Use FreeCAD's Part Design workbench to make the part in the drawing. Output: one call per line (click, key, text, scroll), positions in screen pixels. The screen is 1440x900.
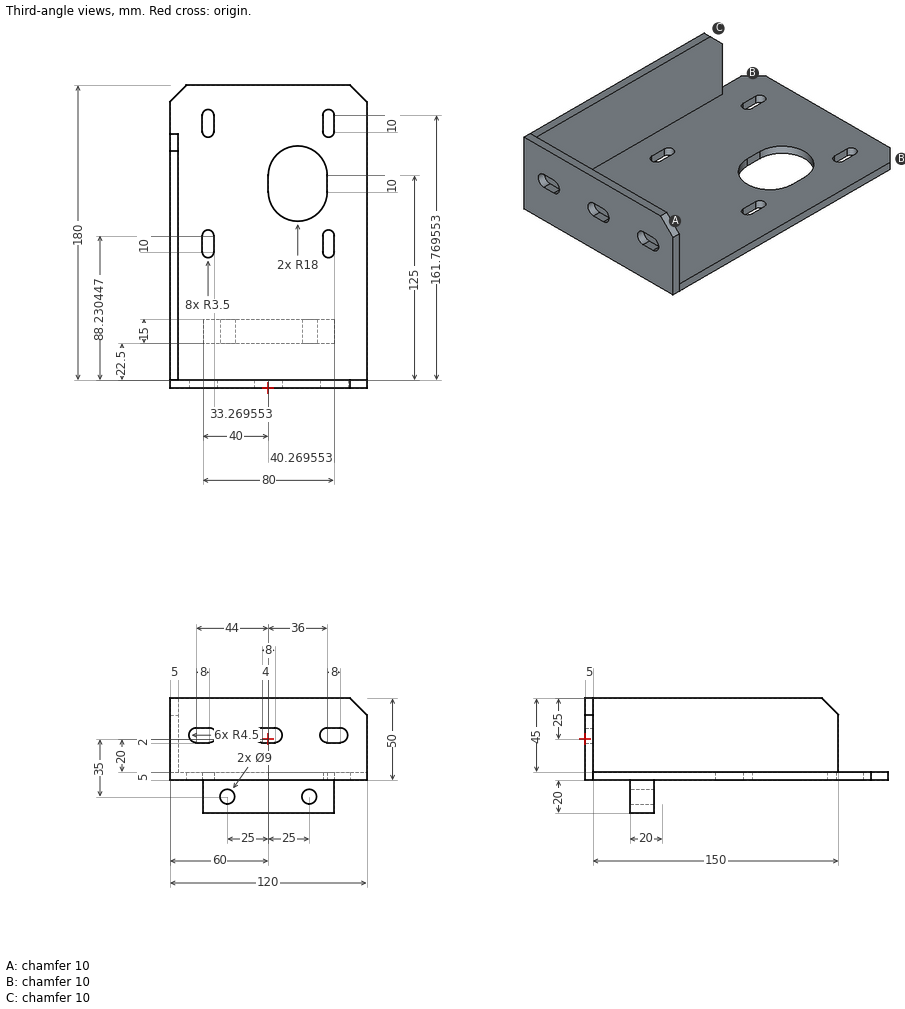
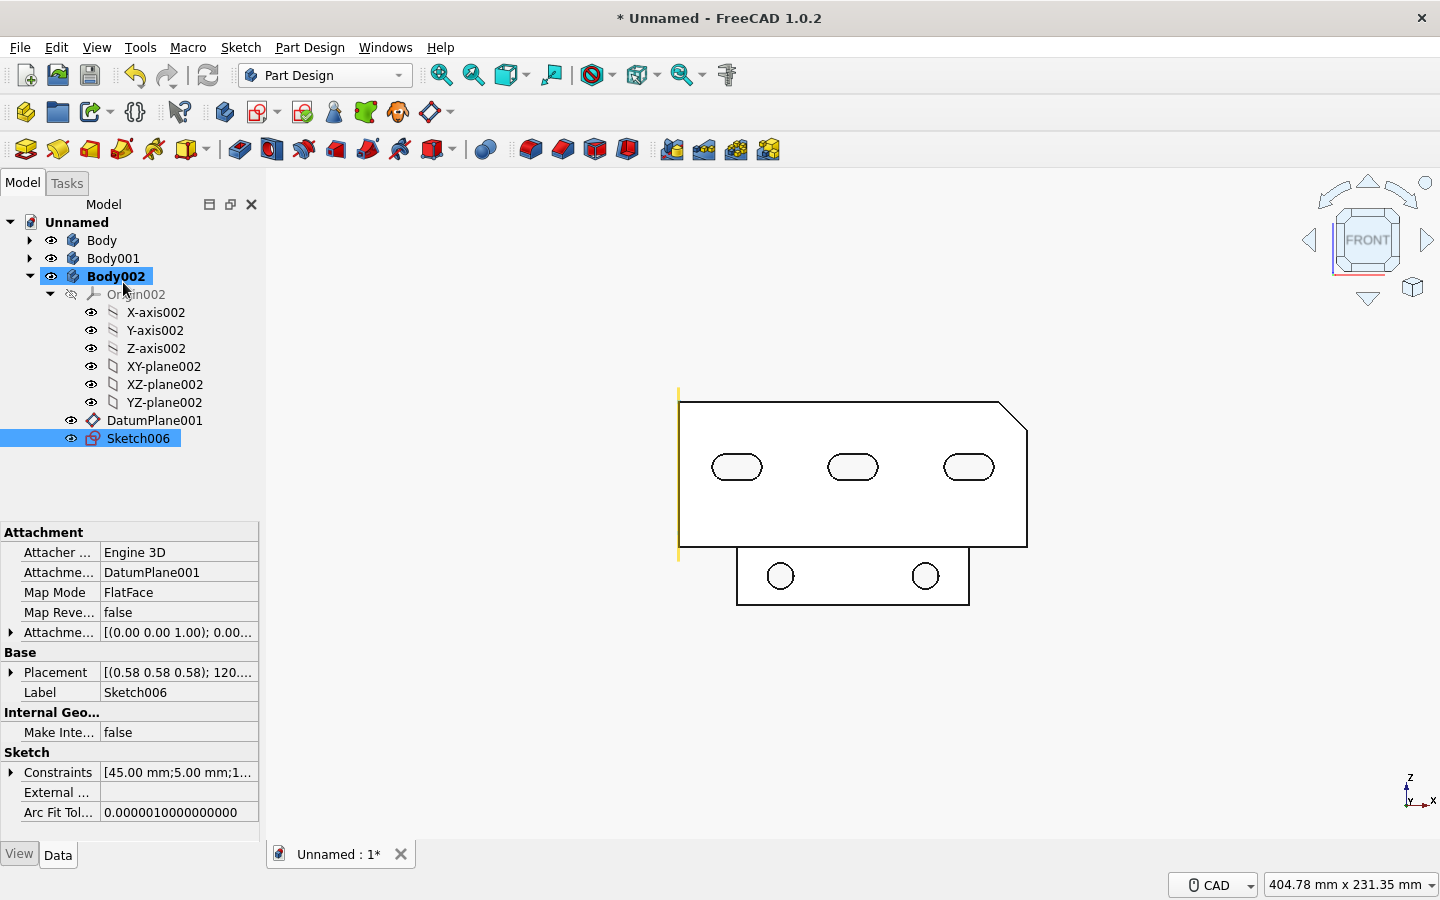
click(26, 150)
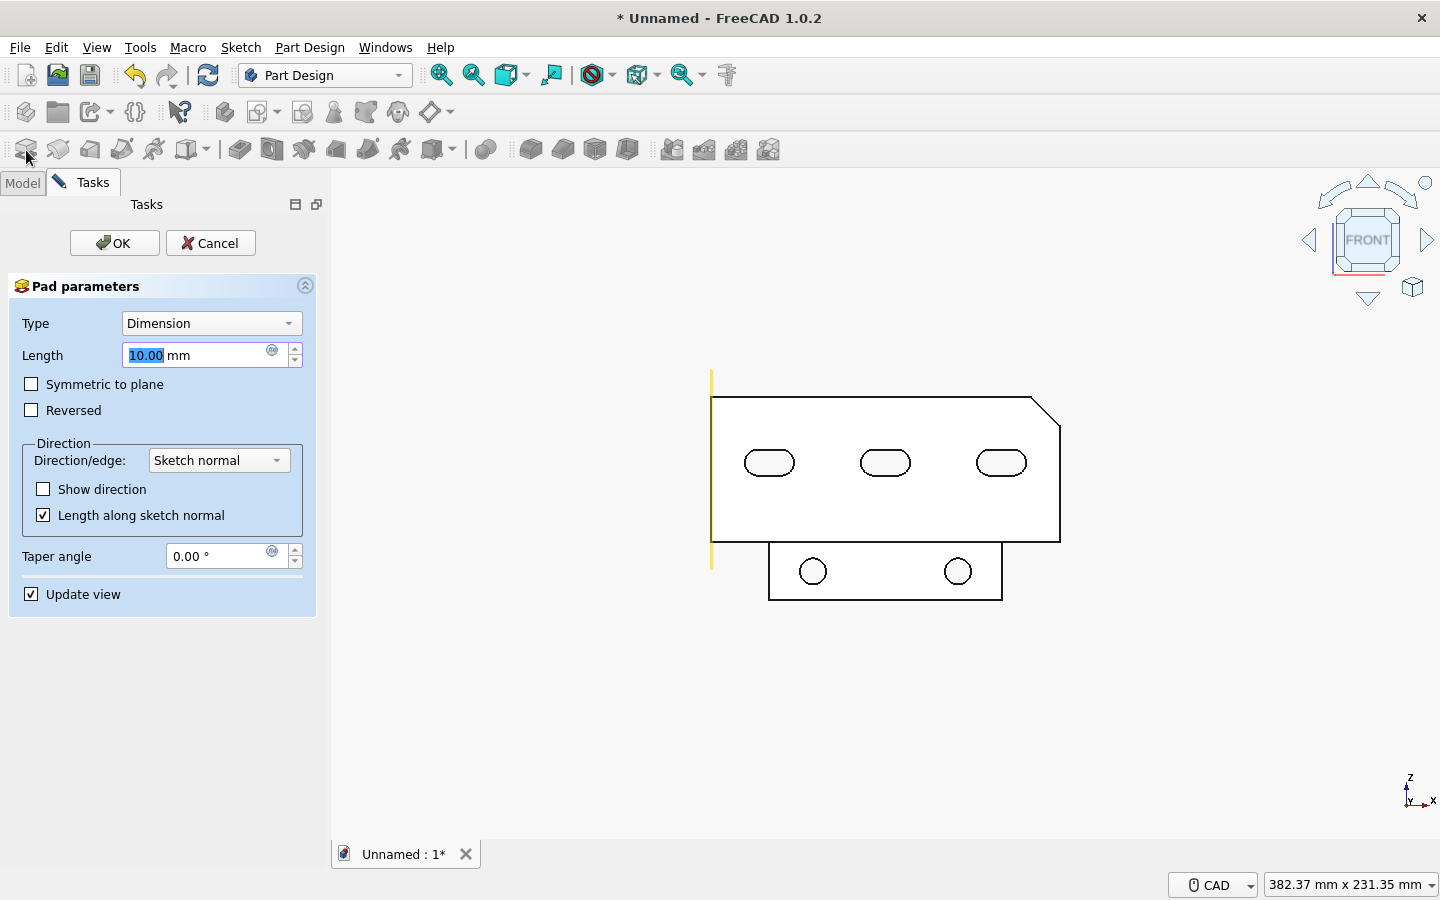
text(5)
key(Tab)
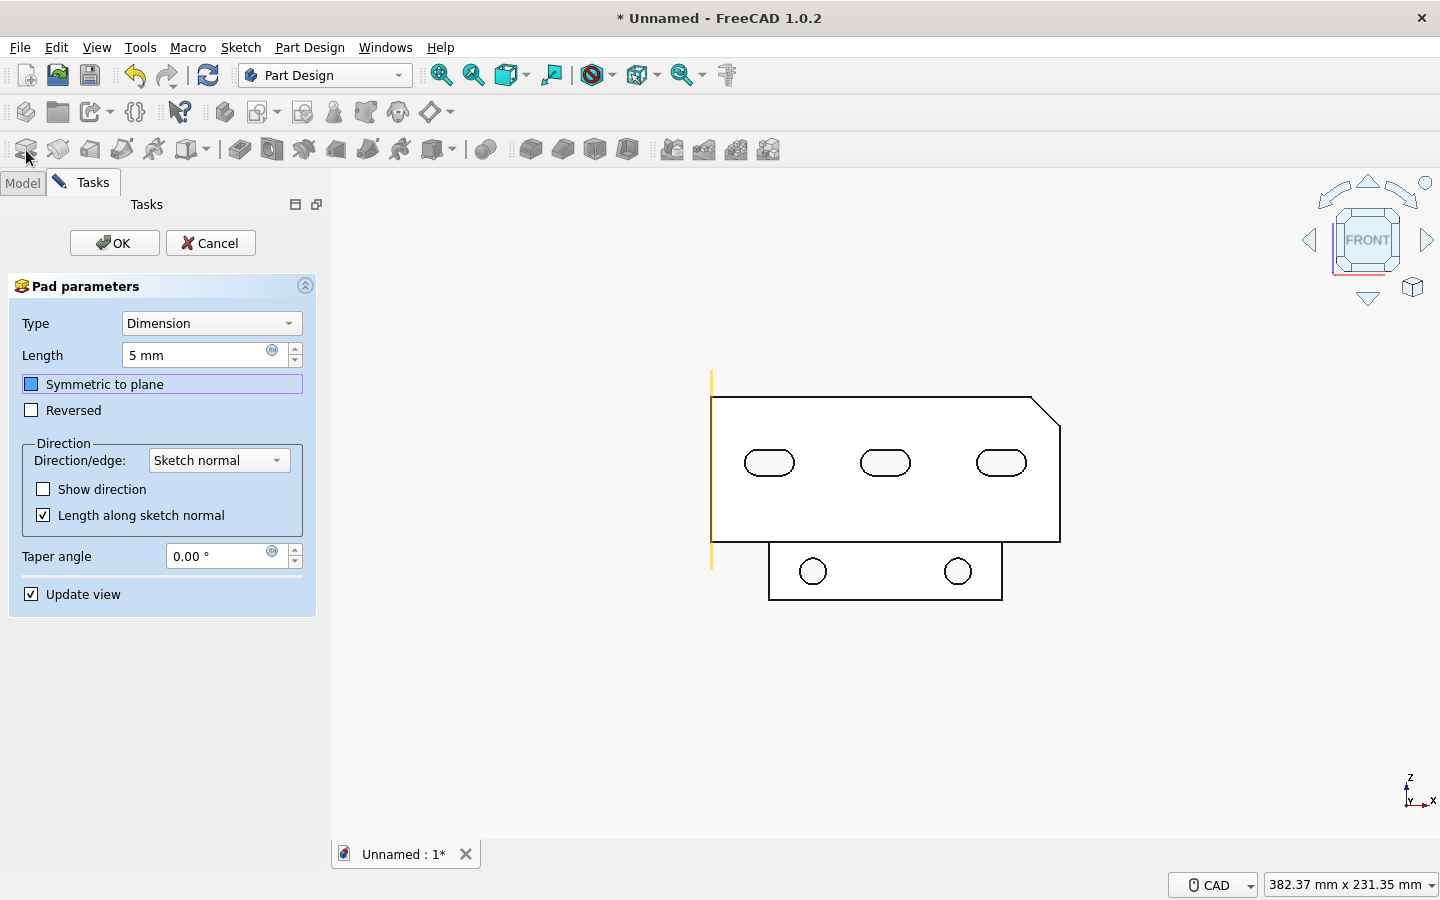
click(115, 243)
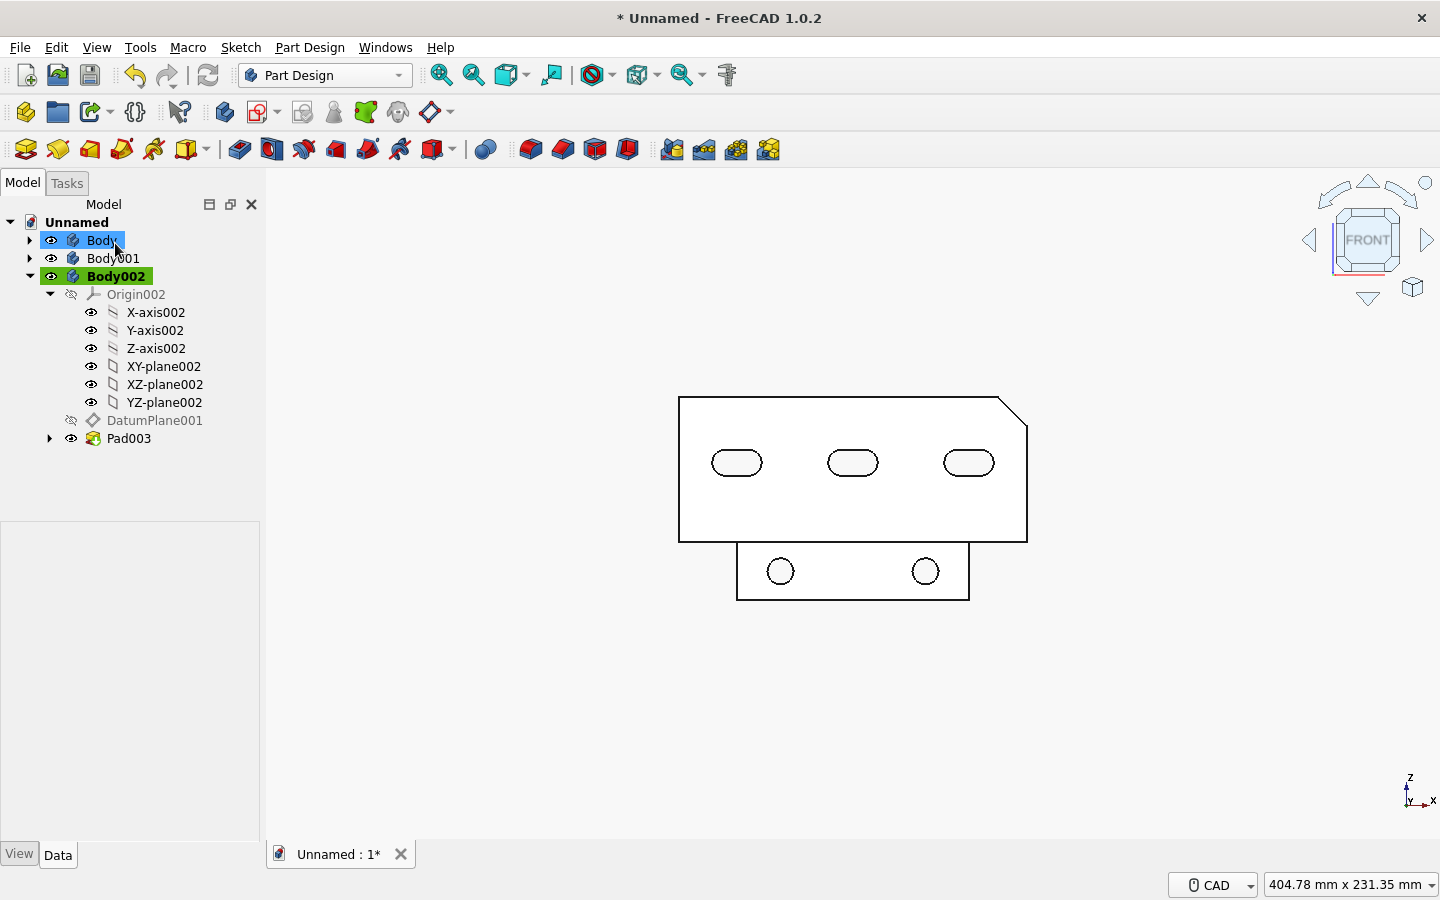
key(v)
key(f)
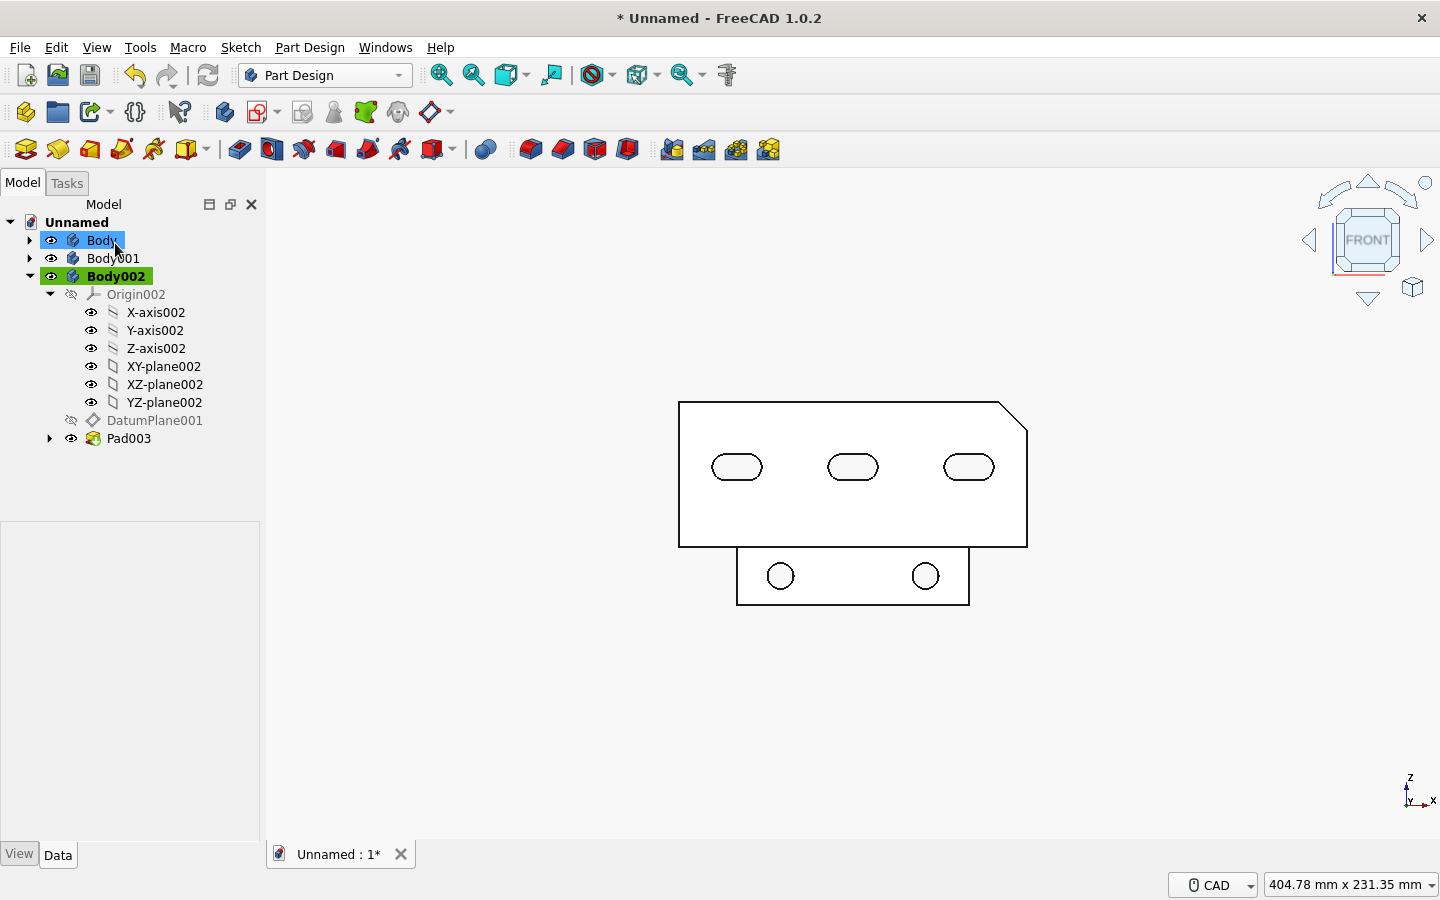
scroll(686, 401, up, 6)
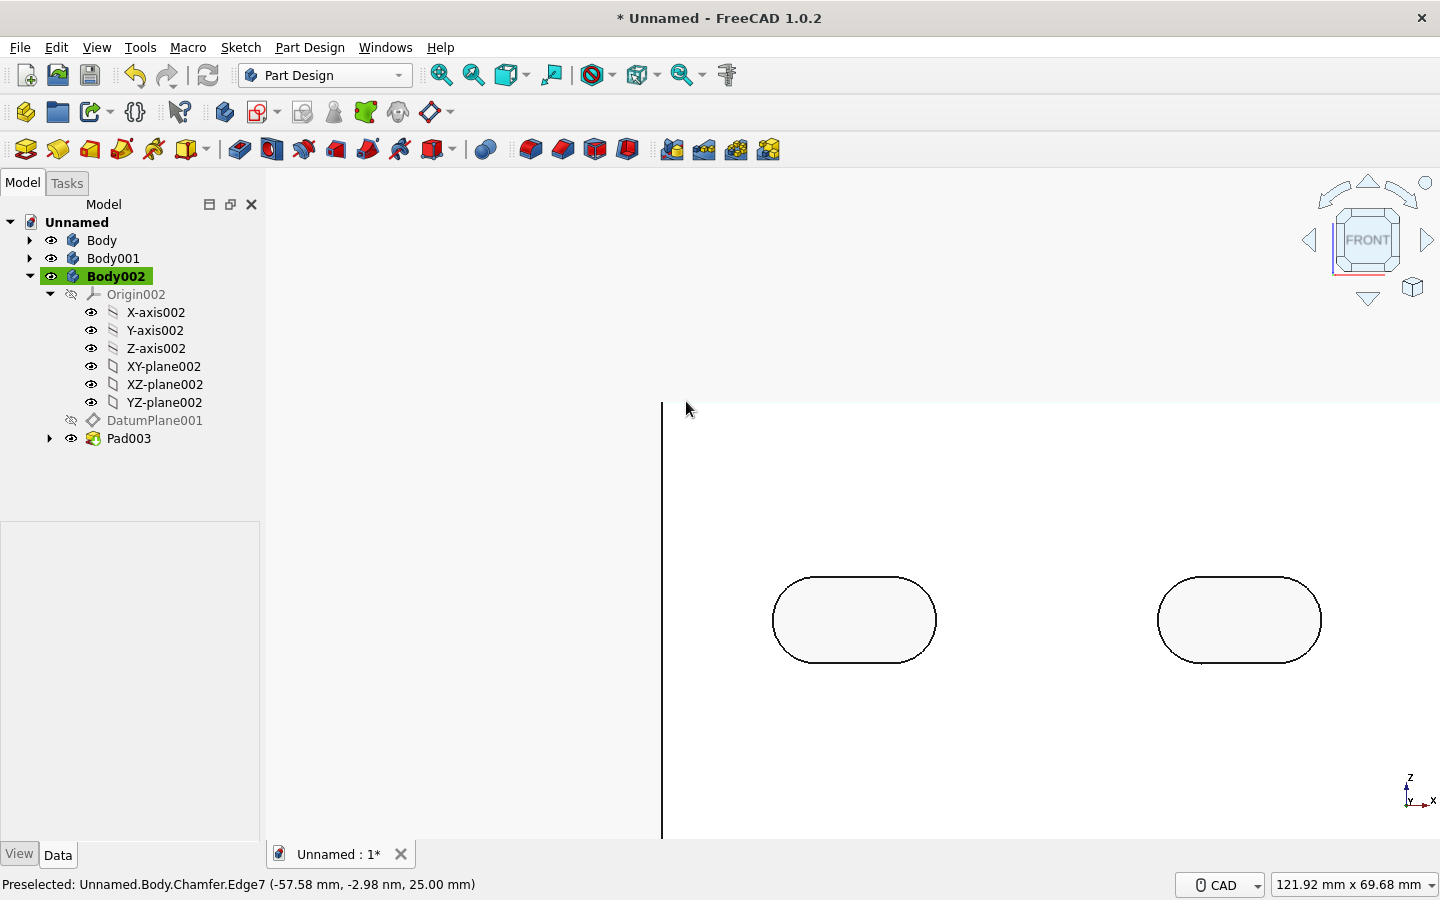
key(v)
key(f)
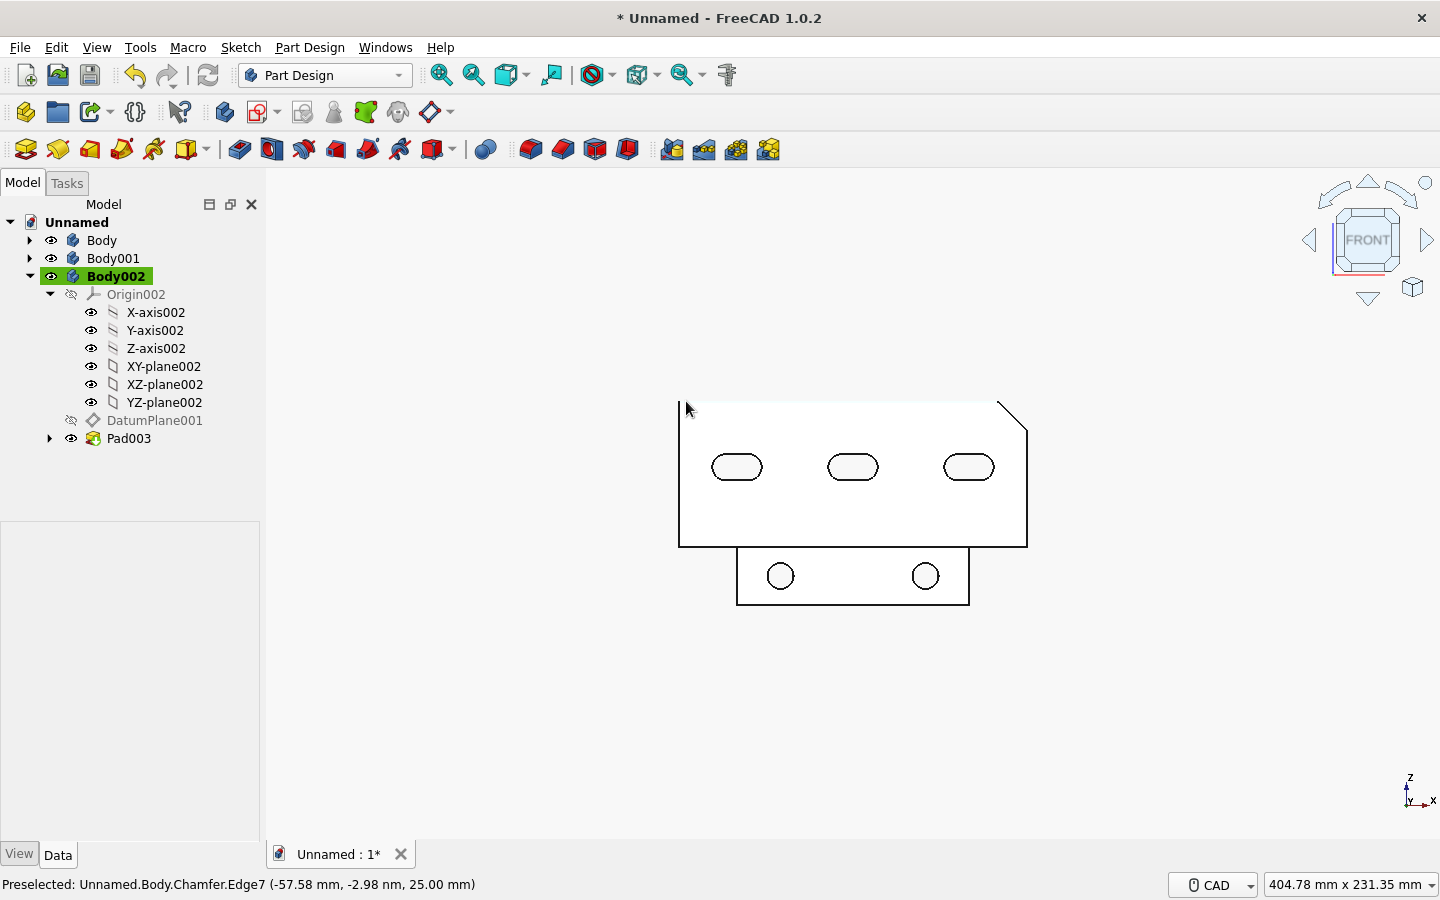
key(0)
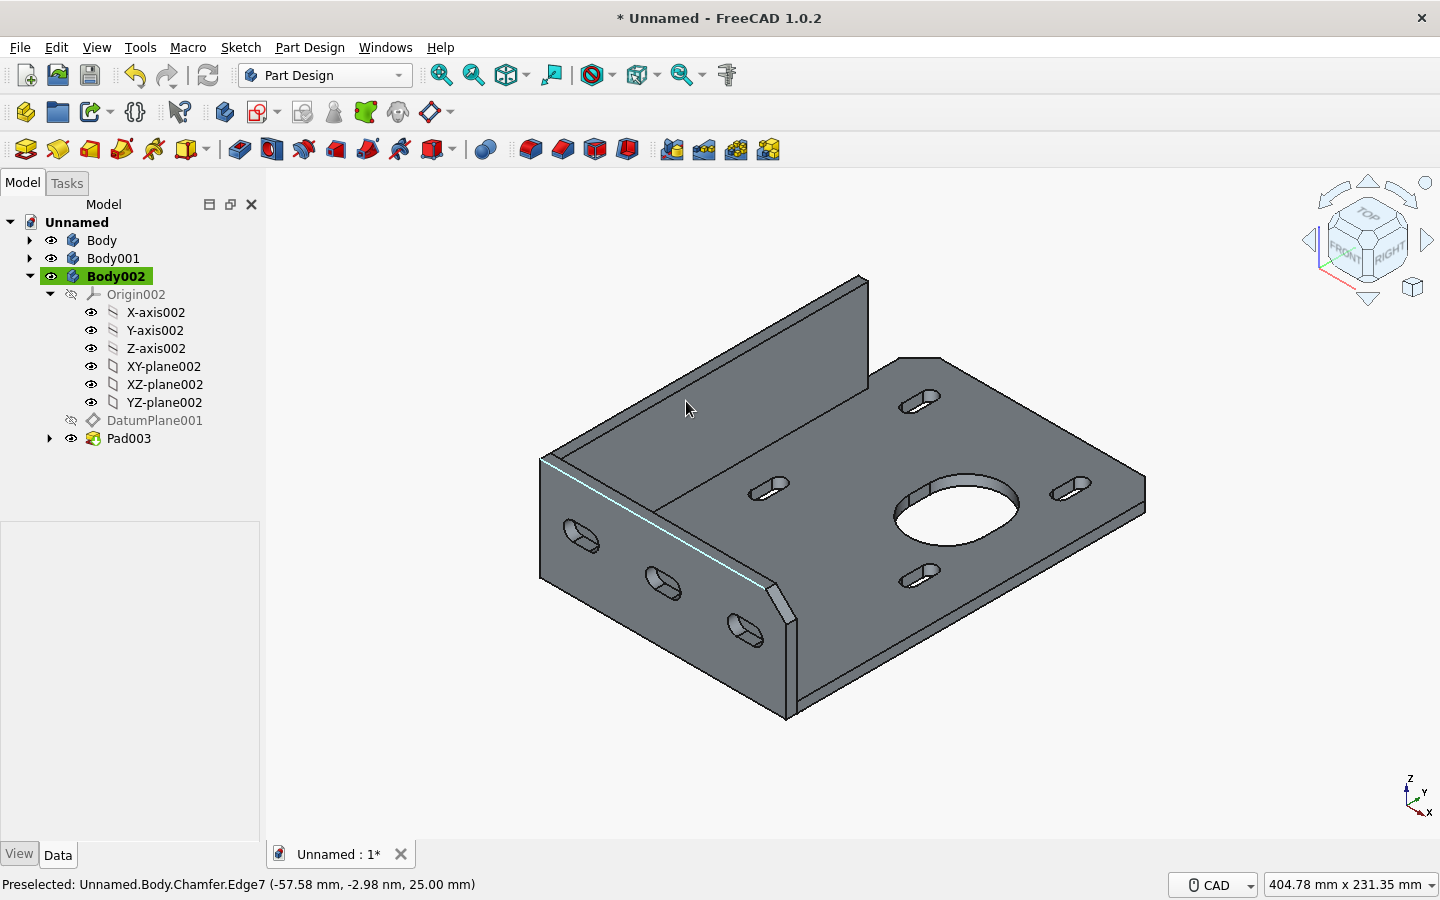
key(v)
key(f)